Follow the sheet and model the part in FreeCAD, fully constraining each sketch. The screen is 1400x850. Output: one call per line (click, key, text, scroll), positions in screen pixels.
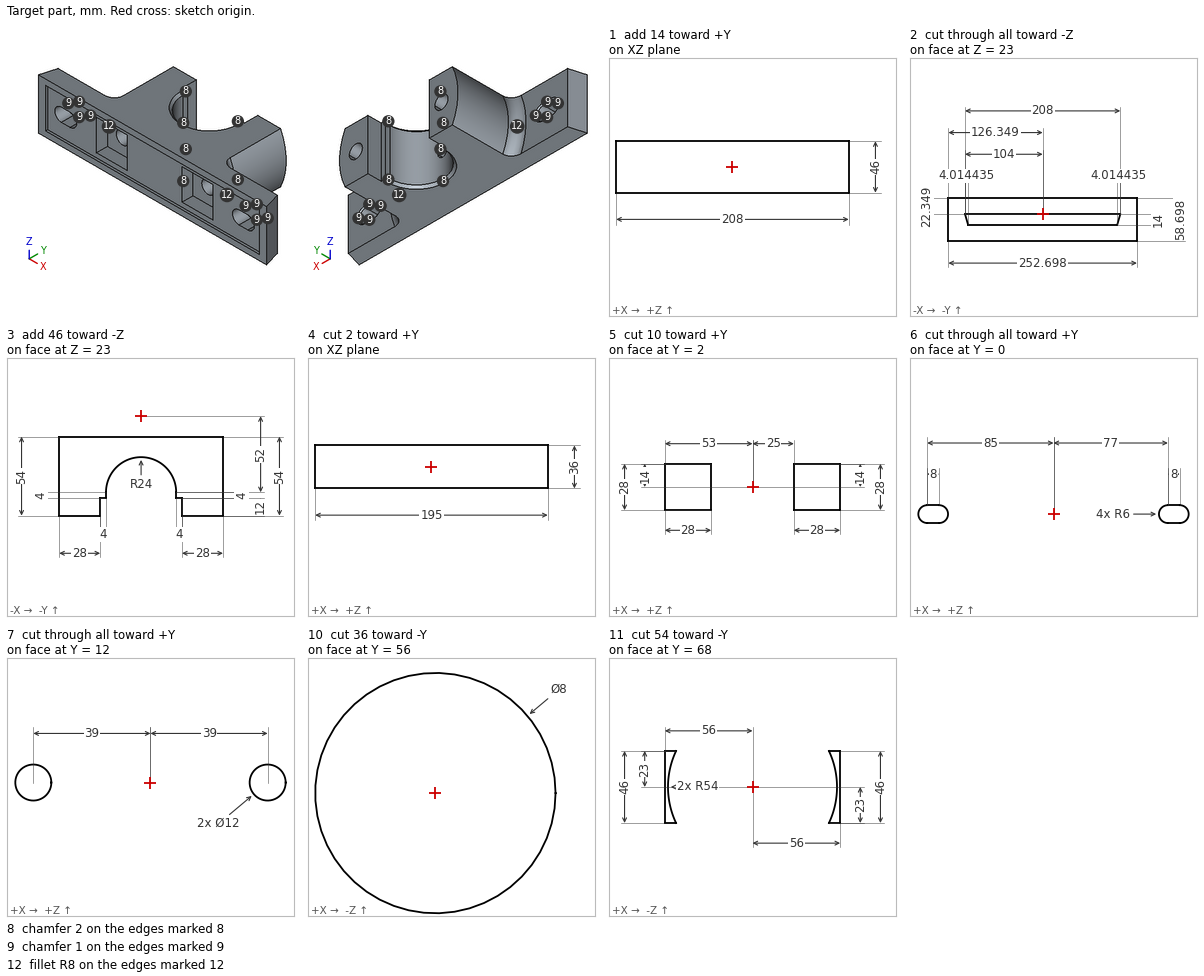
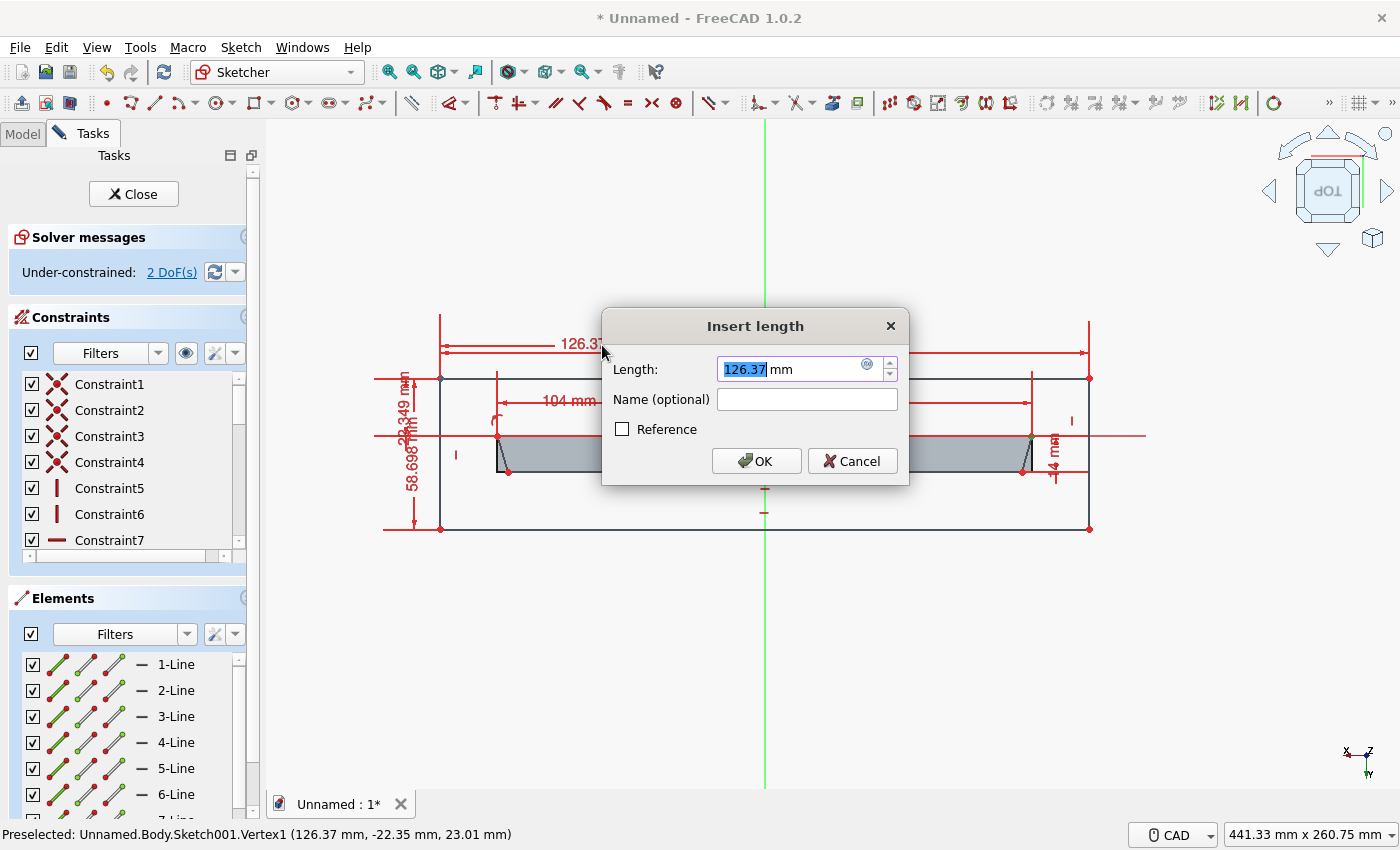
text(126.349)
key(Return)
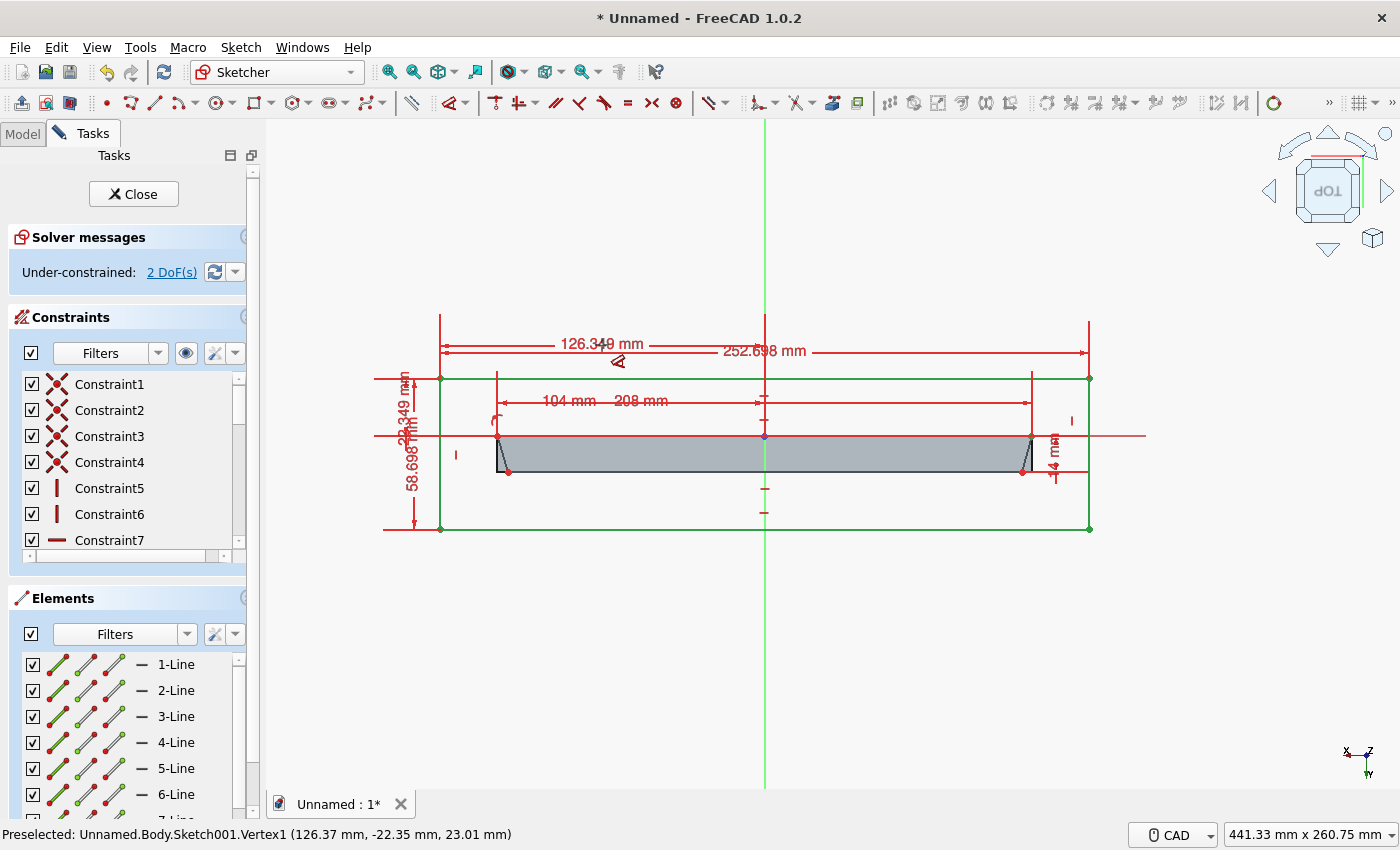
scroll(505, 461, up, 7)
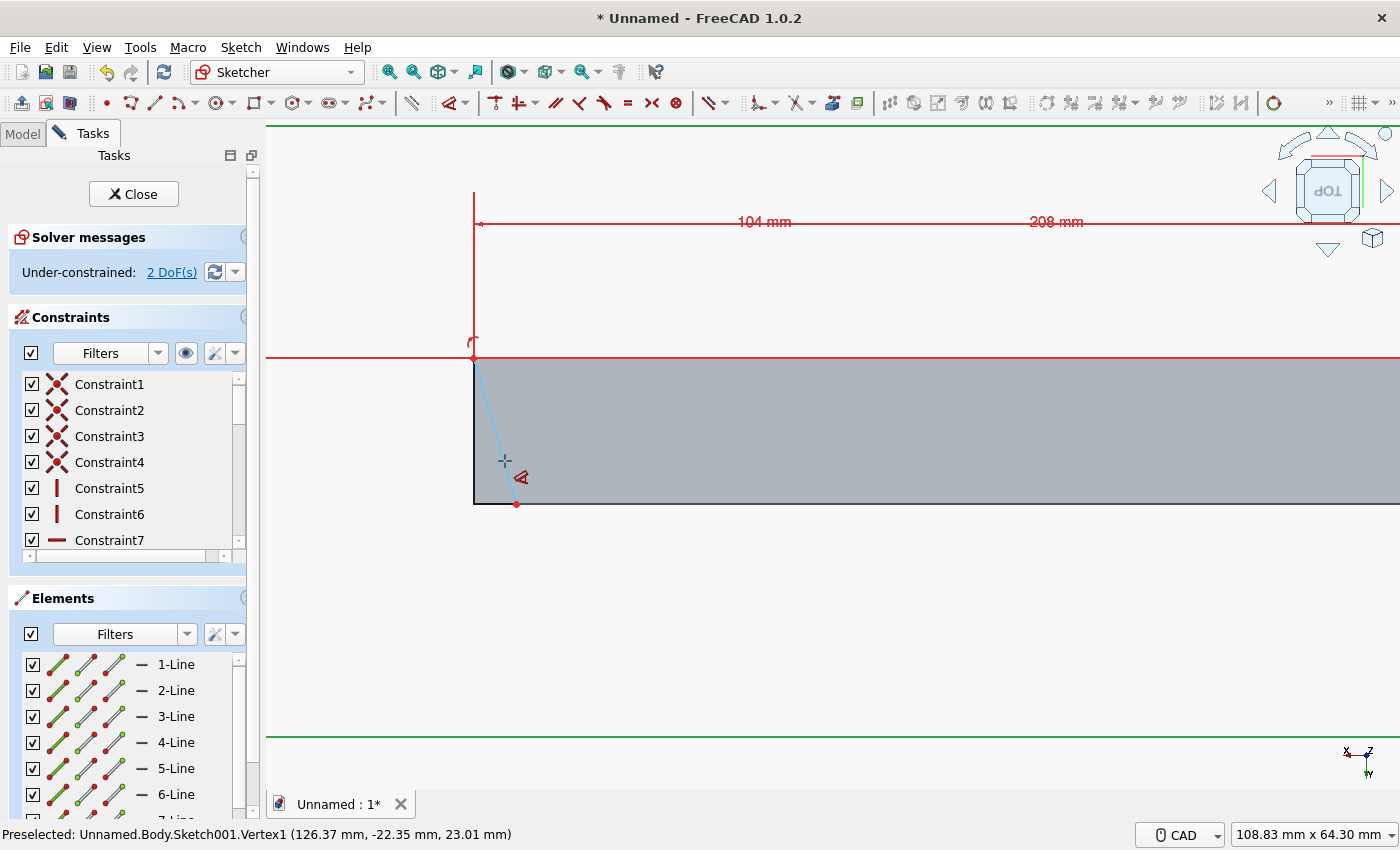
click(504, 461)
click(495, 538)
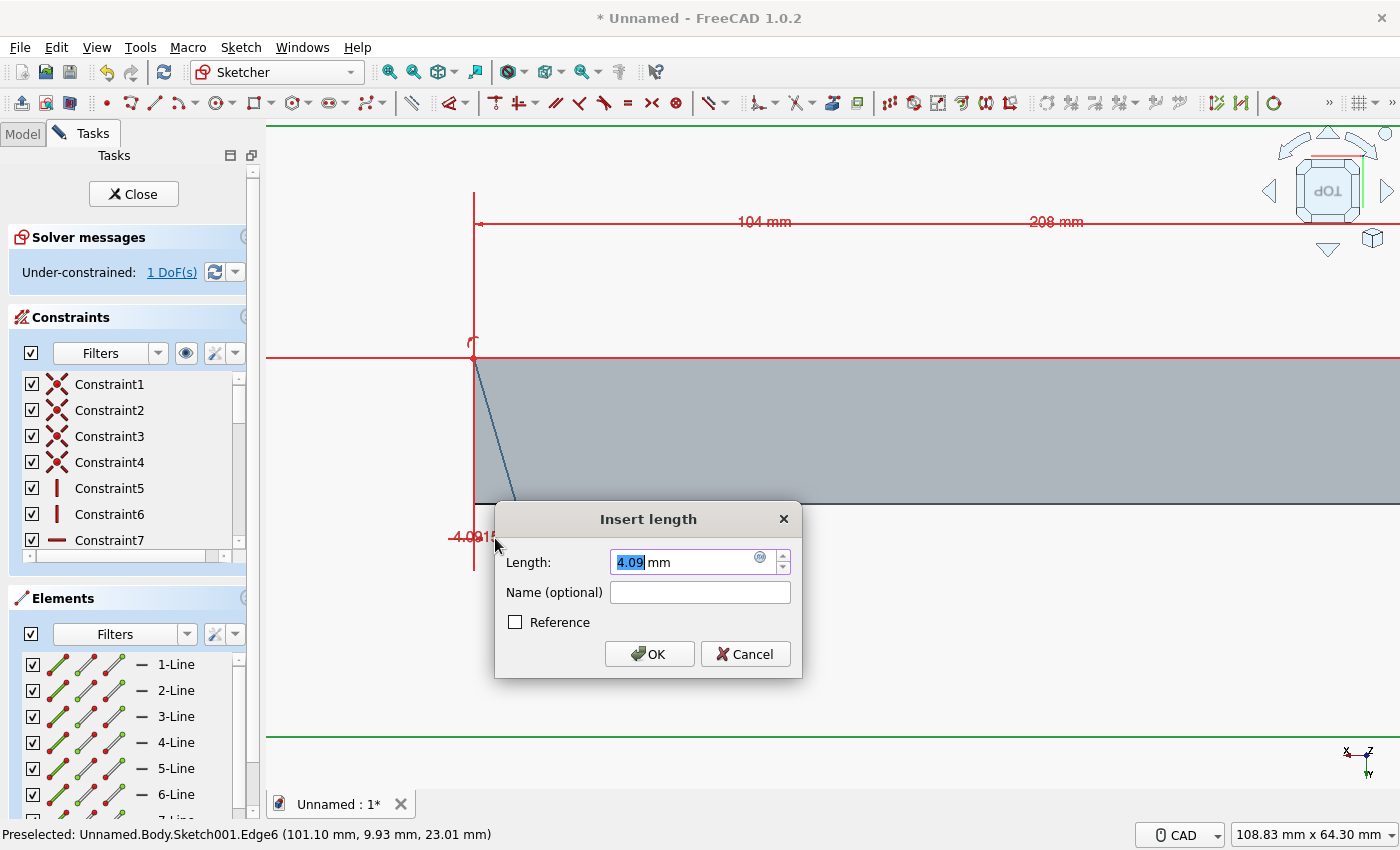
text(4.014435)
key(Return)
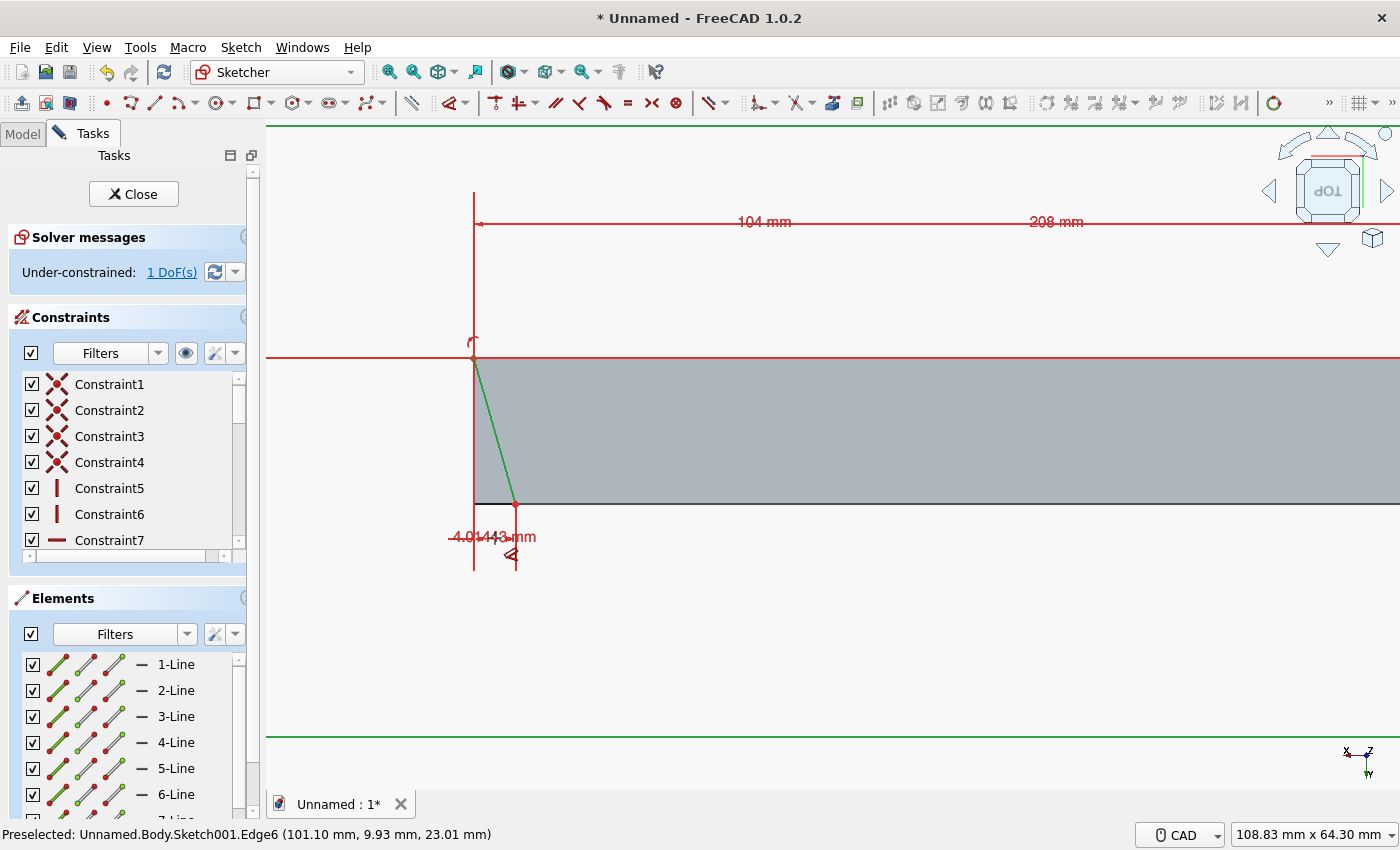
scroll(505, 461, down, 7)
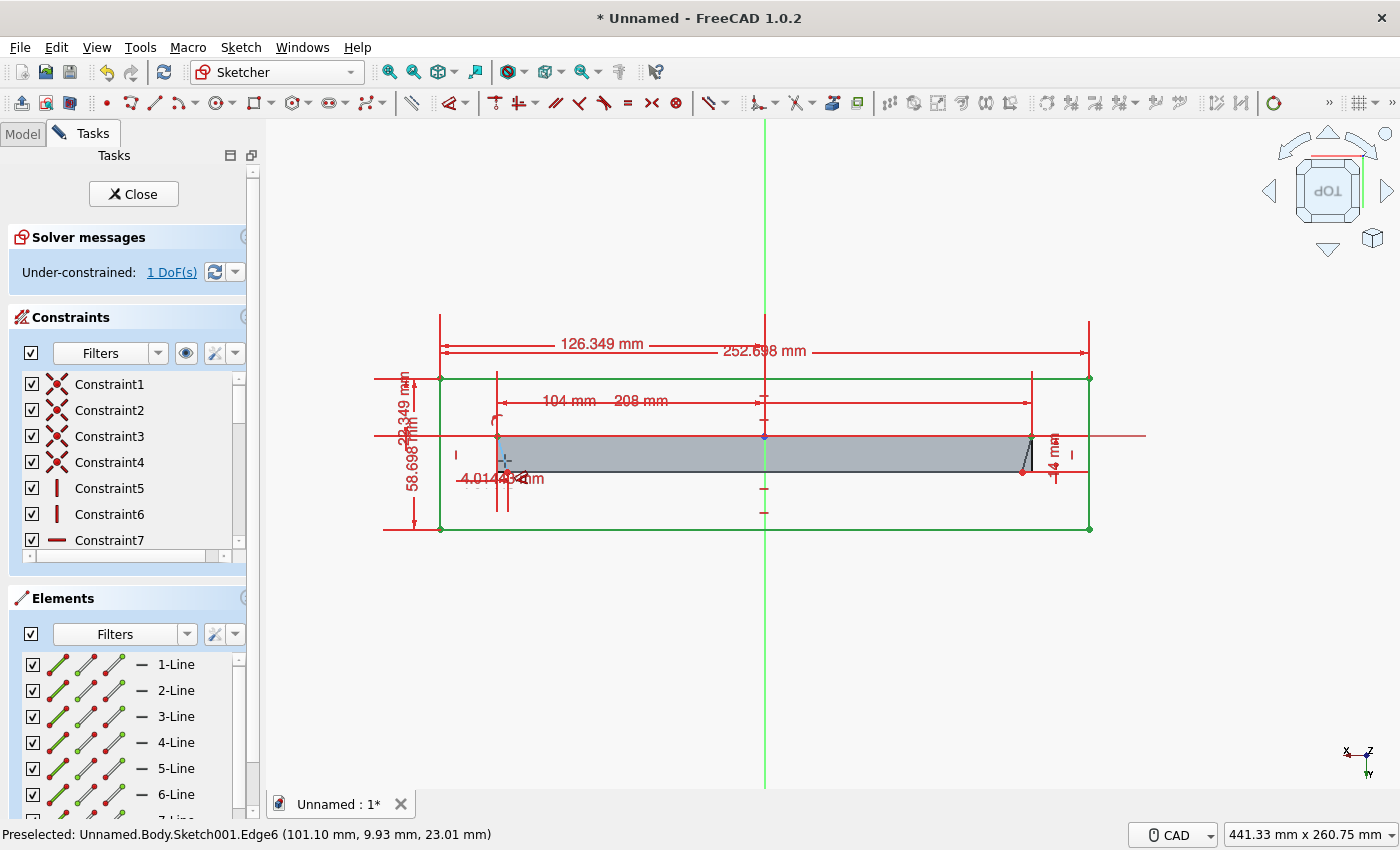
scroll(1029, 447, up, 7)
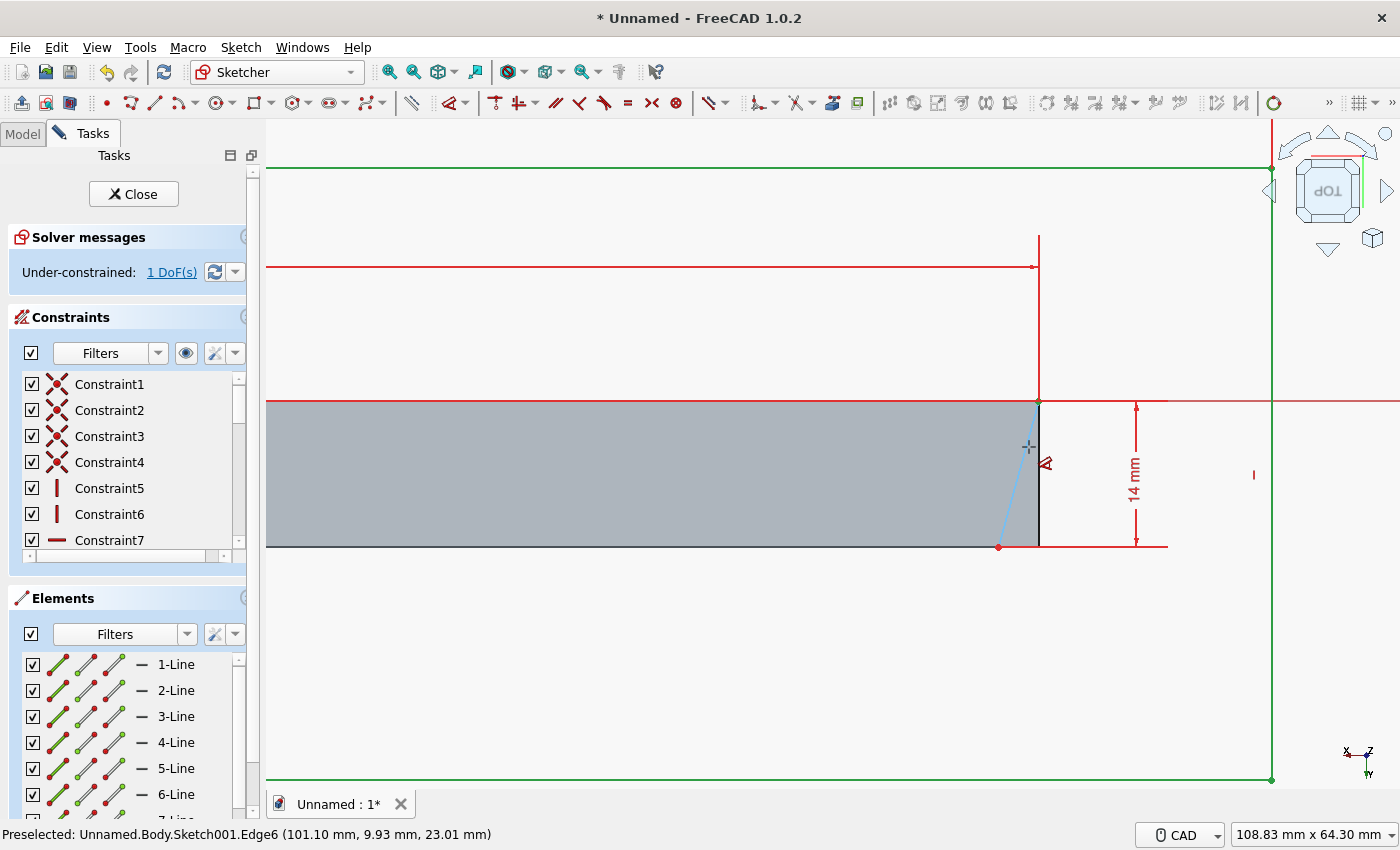
click(1027, 445)
click(1019, 581)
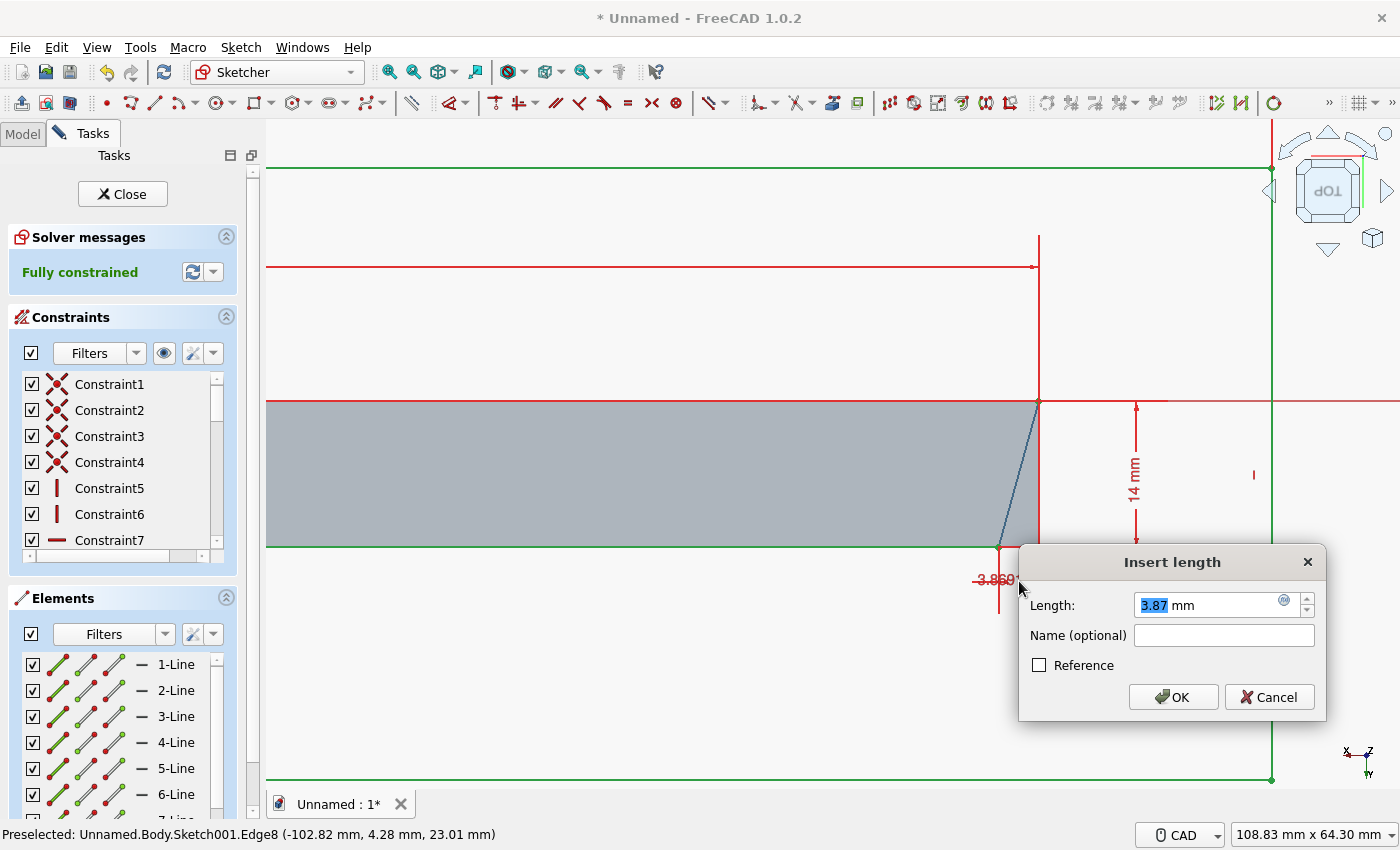
text(4.014435)
key(Return)
key(Escape)